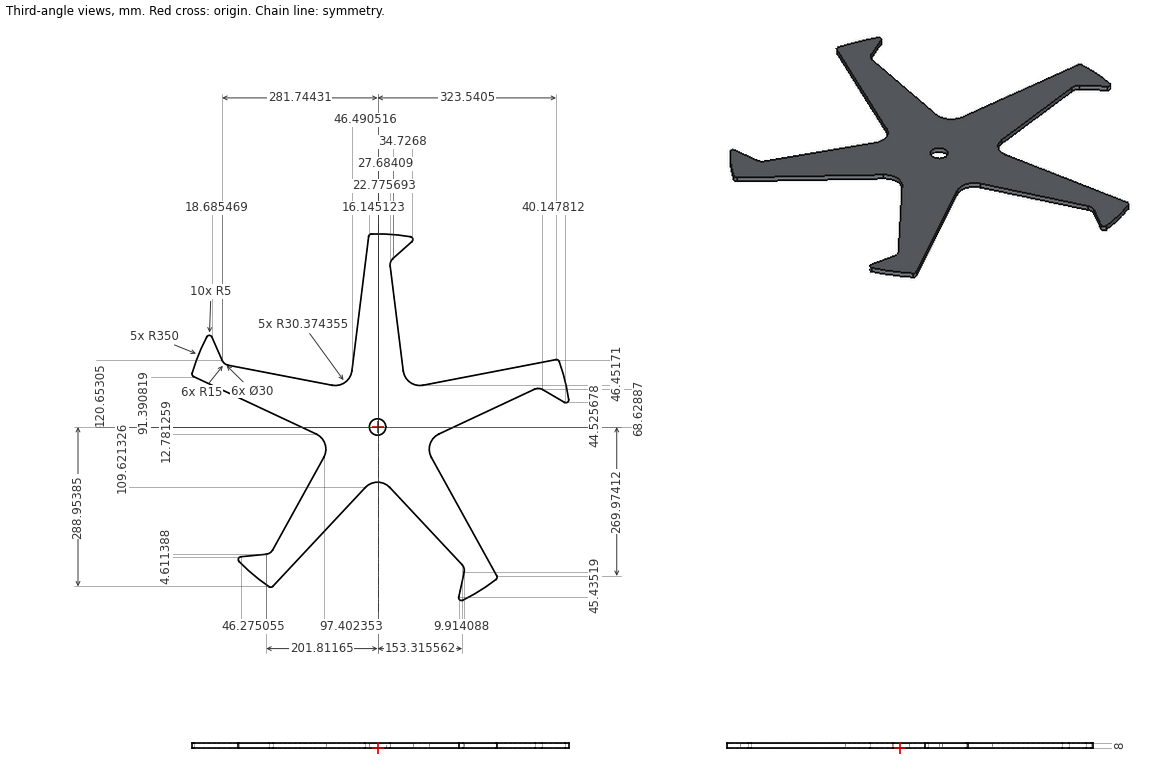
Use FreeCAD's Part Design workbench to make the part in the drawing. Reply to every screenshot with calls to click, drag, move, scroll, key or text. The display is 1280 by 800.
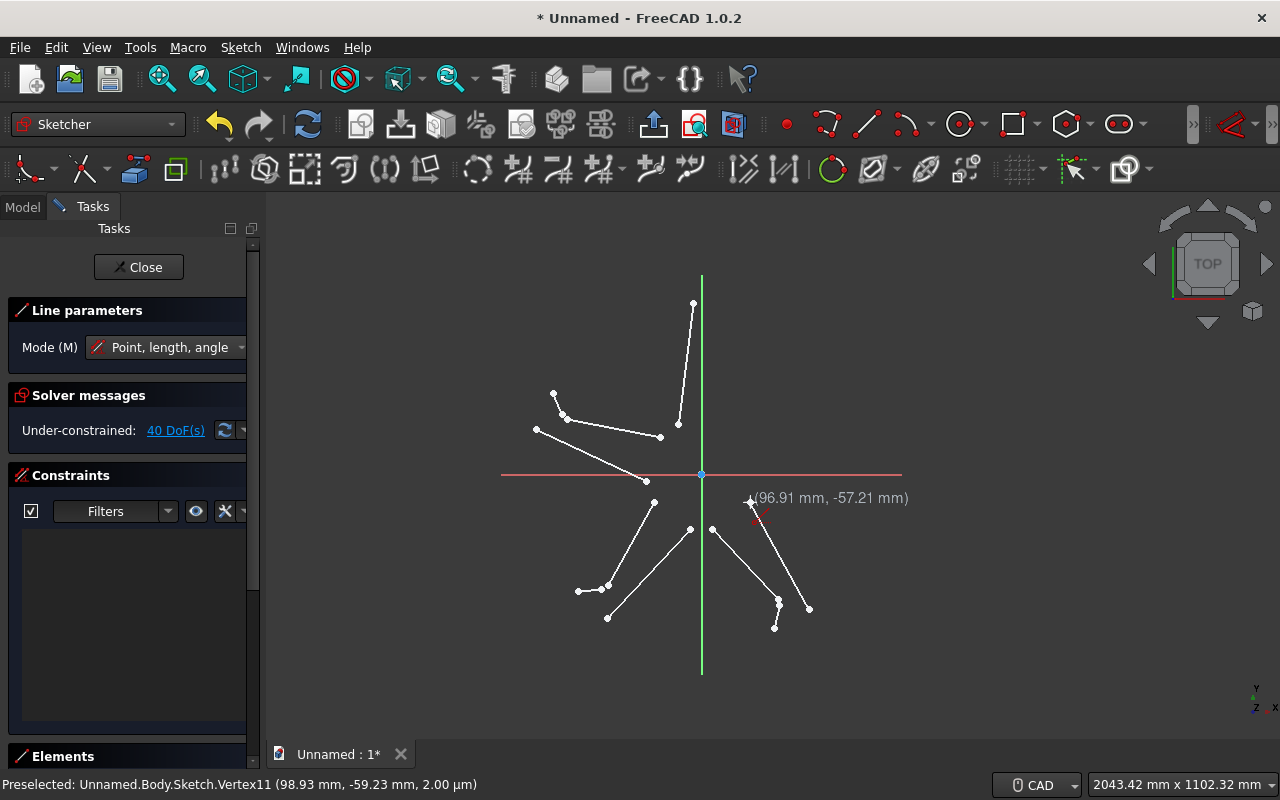
scroll(757, 481, up, 5)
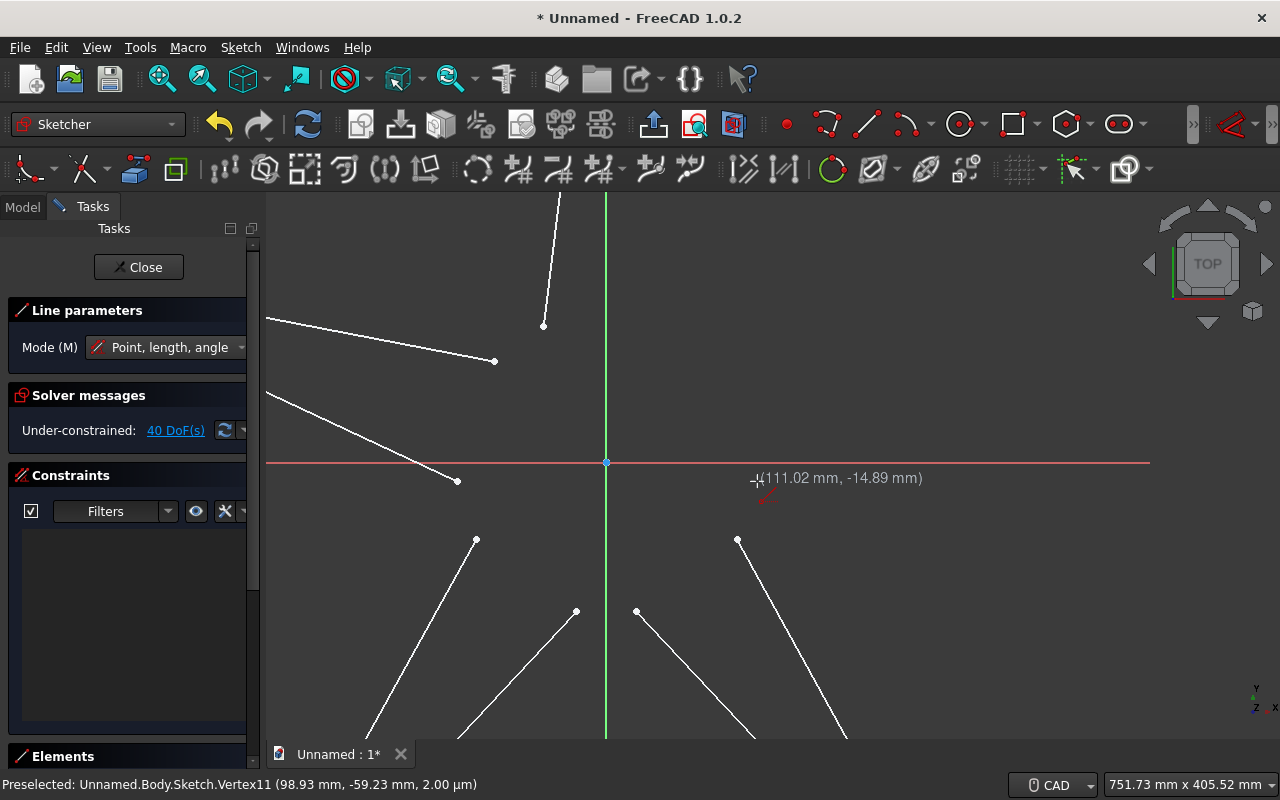
click(756, 480)
click(991, 370)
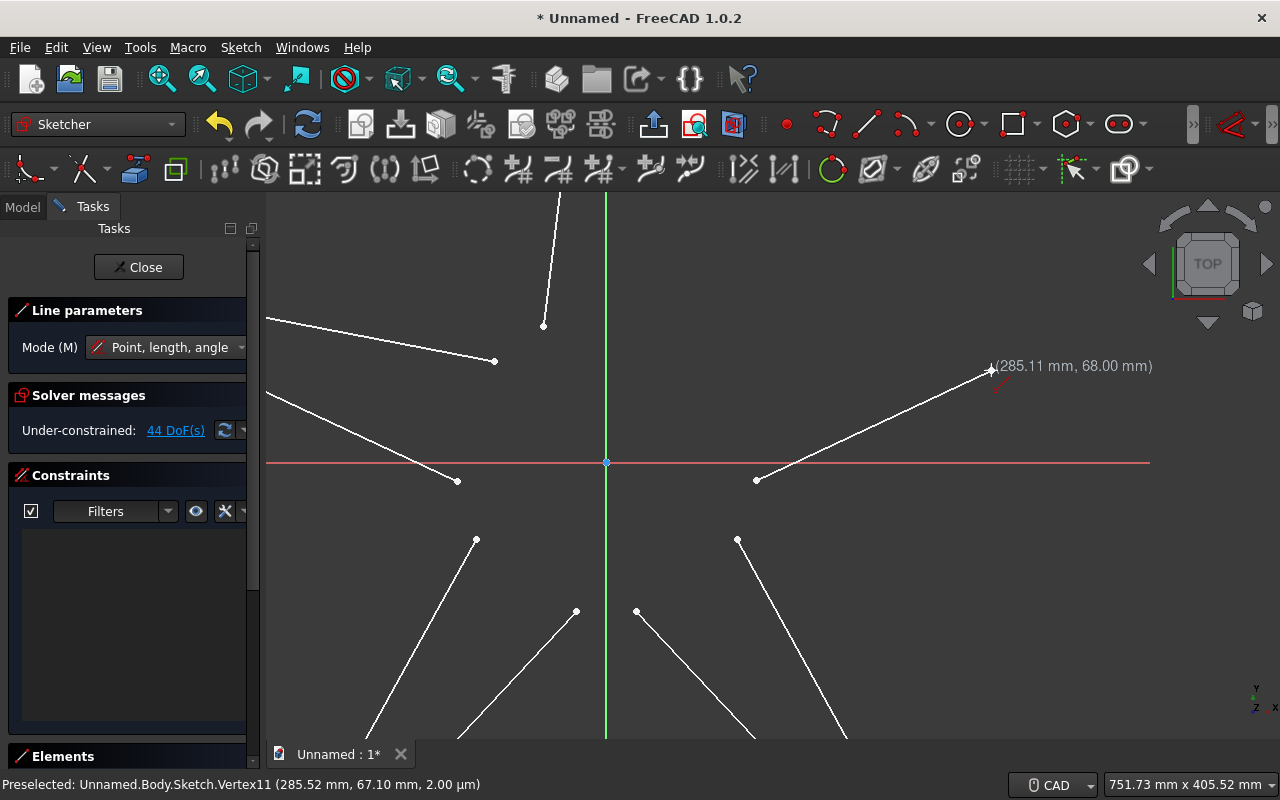
click(1010, 371)
click(1064, 403)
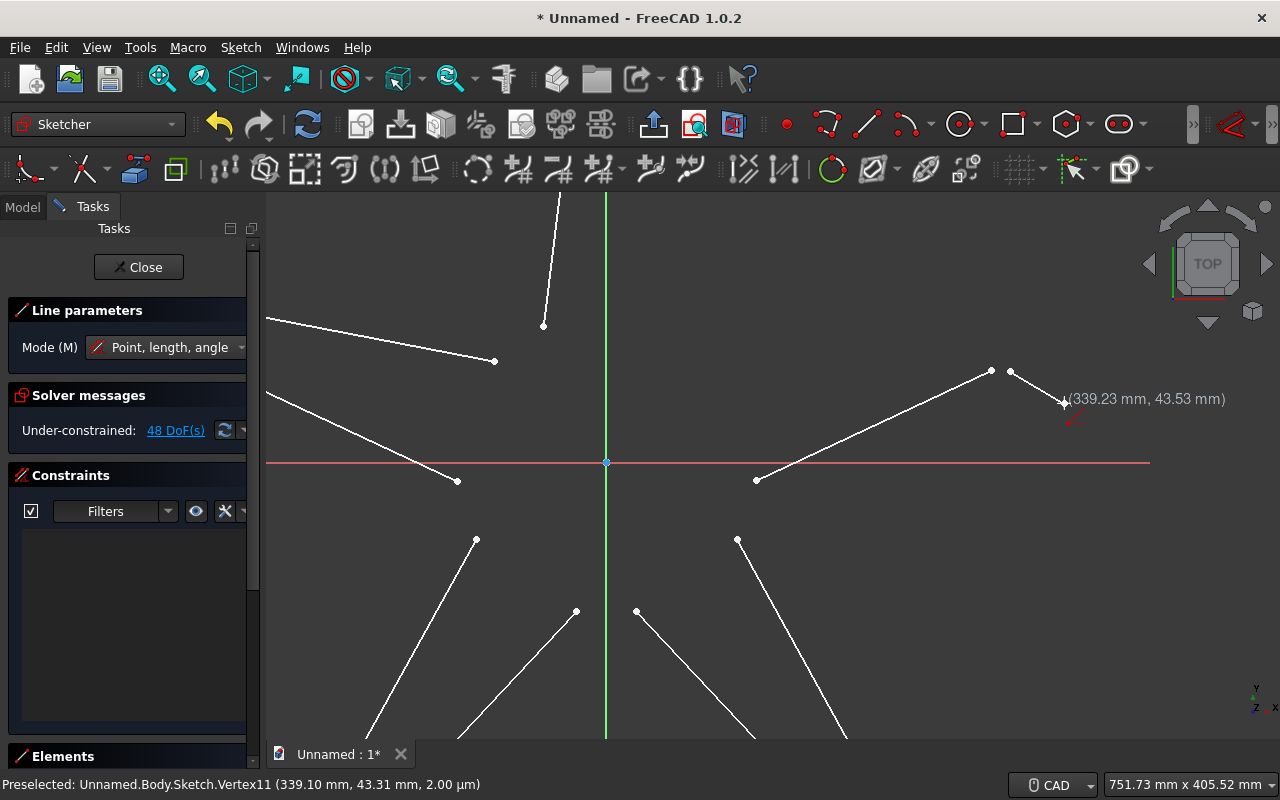
click(1043, 298)
click(718, 361)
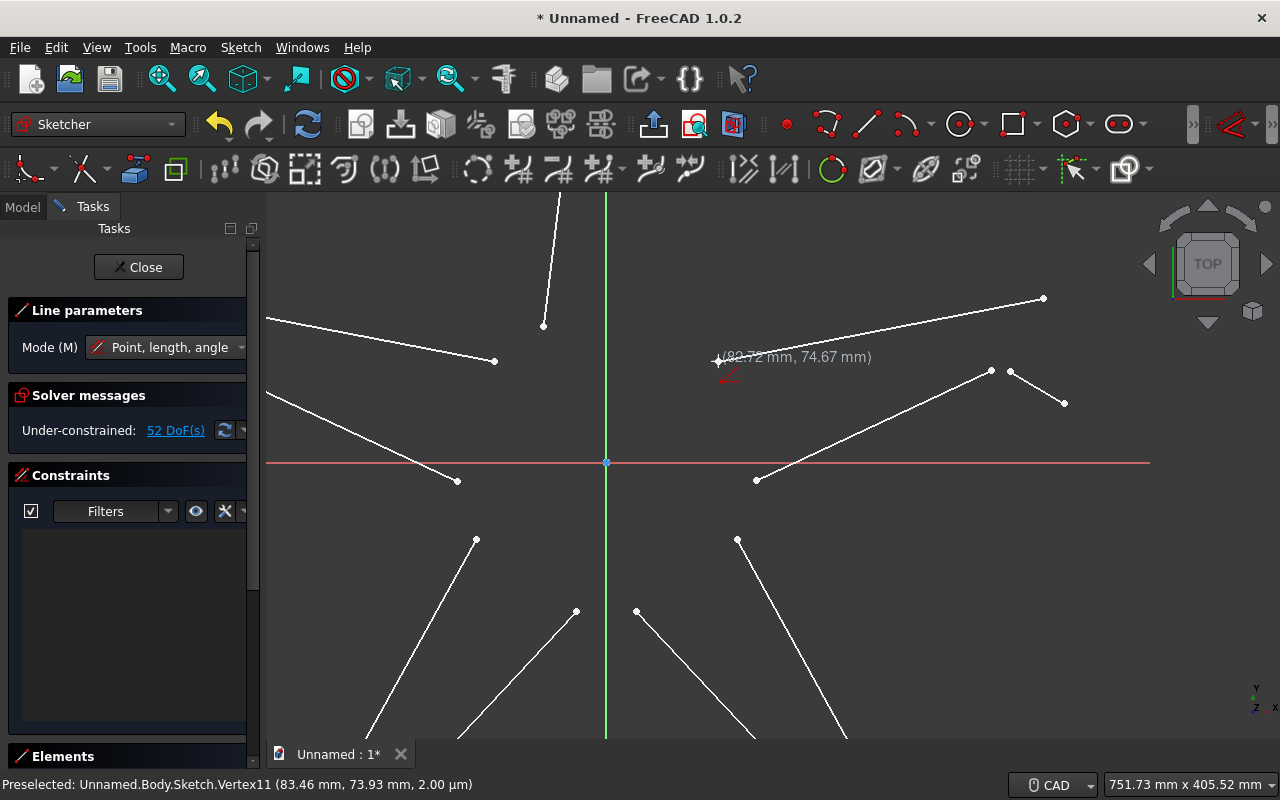
click(669, 326)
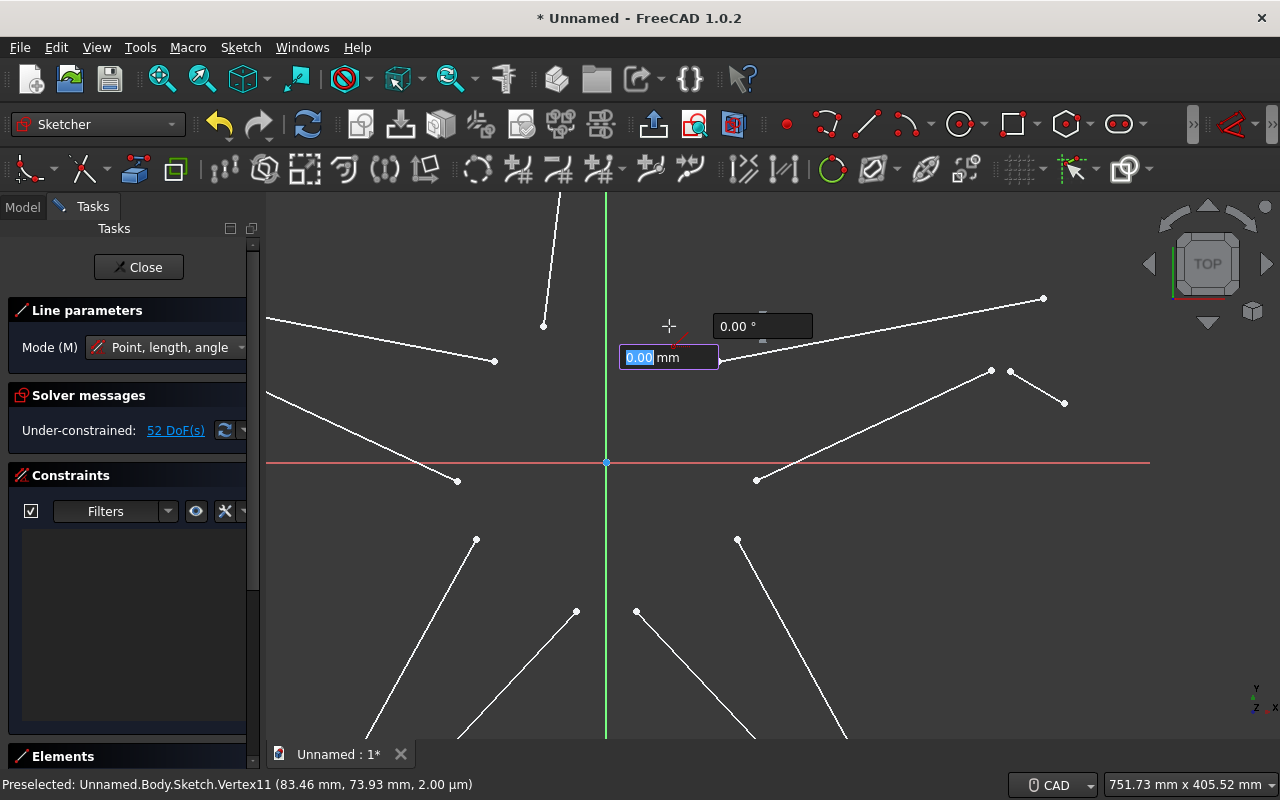
scroll(758, 481, down, 5)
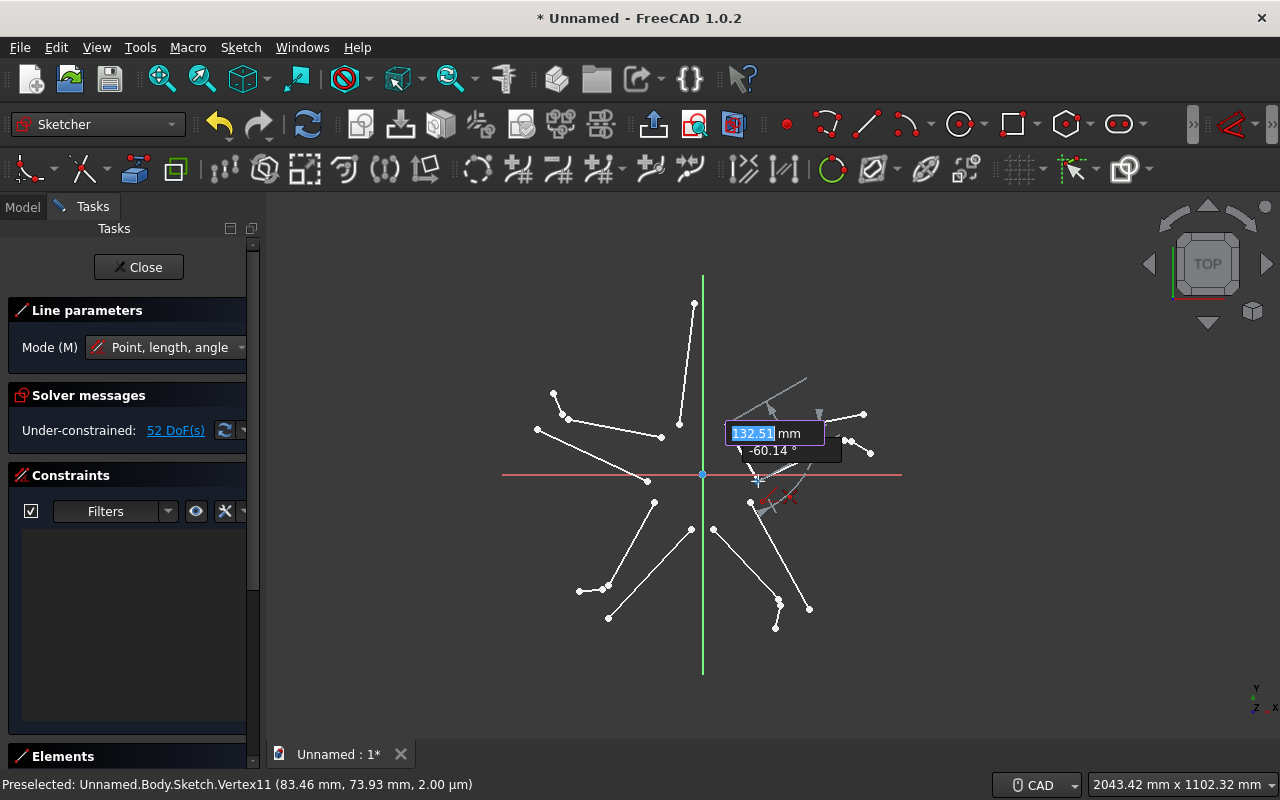
scroll(714, 330, up, 2)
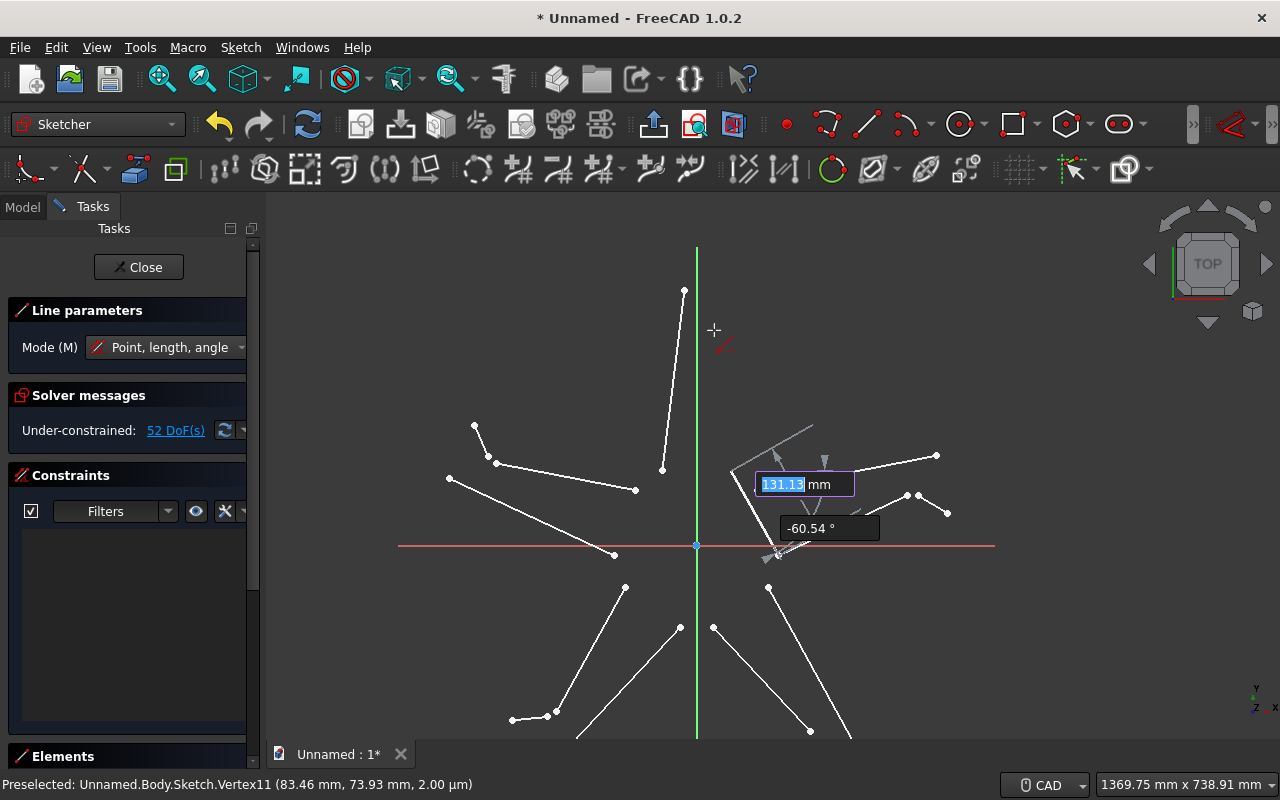
click(714, 329)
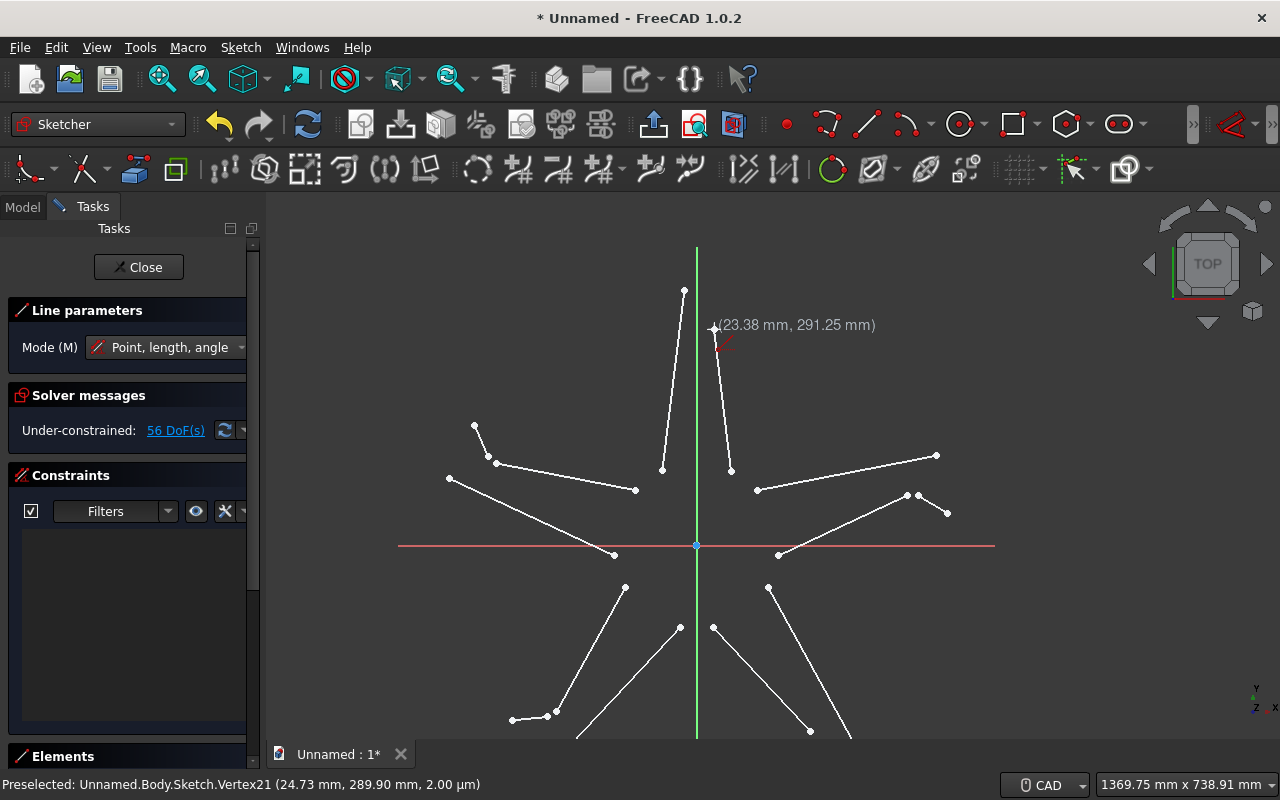
scroll(717, 320, up, 3)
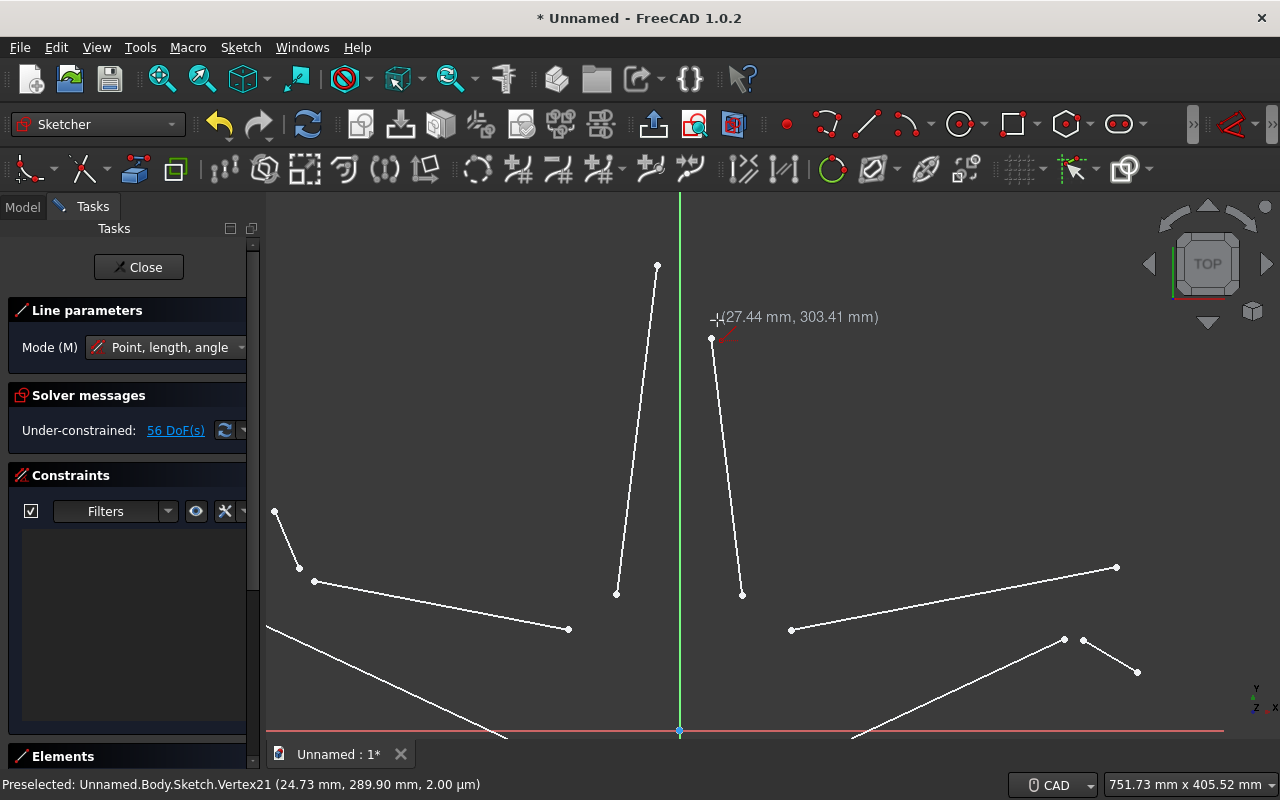
click(717, 319)
click(764, 277)